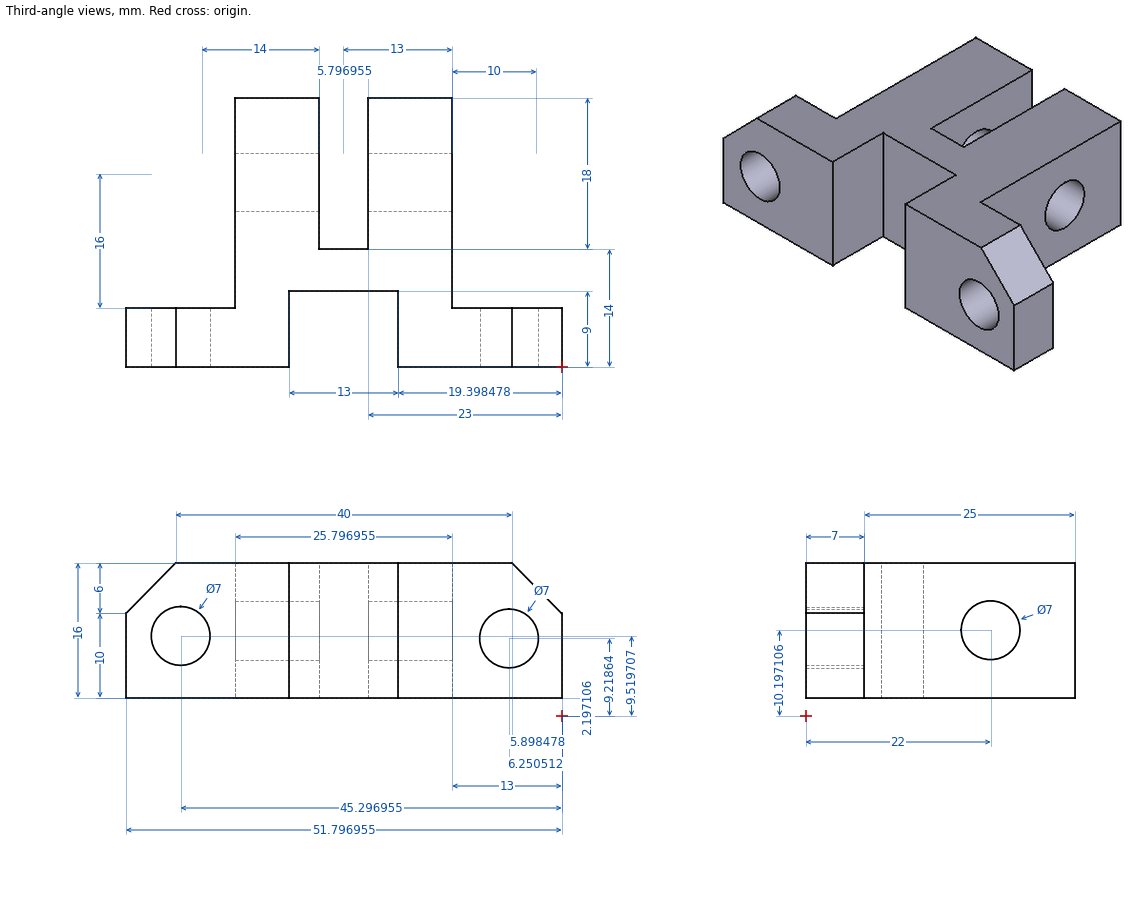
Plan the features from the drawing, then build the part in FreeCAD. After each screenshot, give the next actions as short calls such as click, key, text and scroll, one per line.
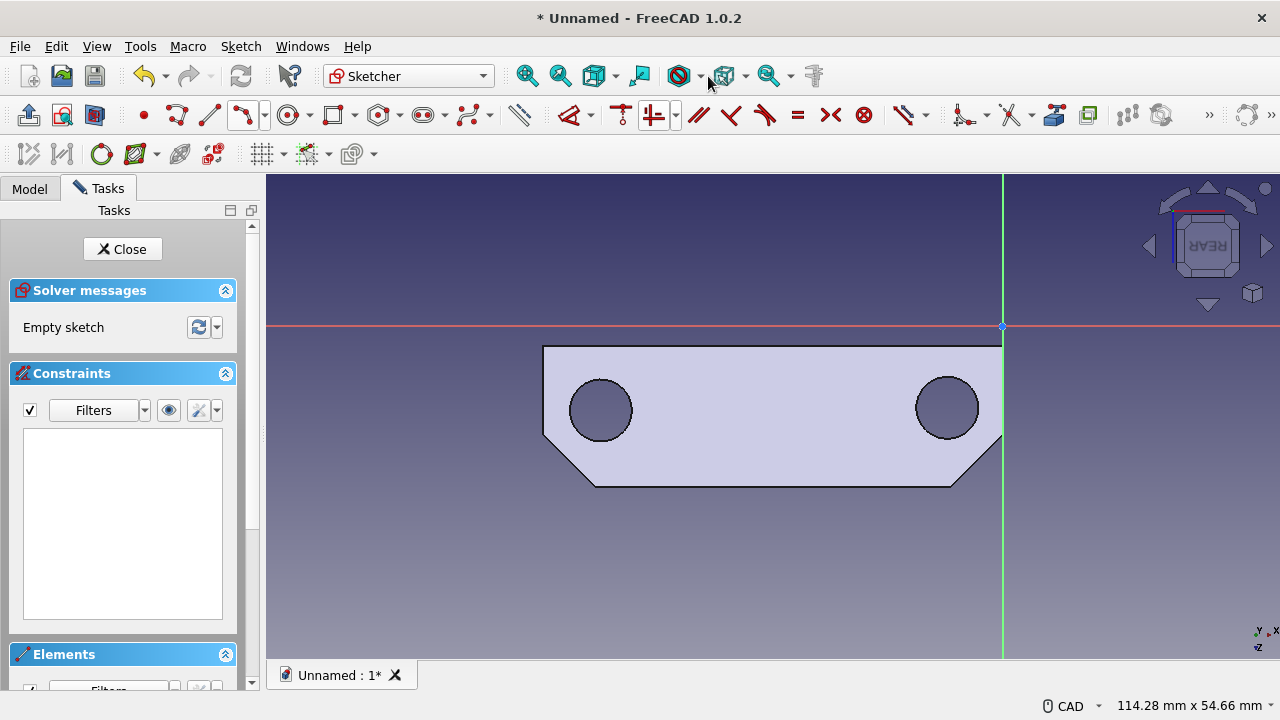
scroll(984, 395, up, 3)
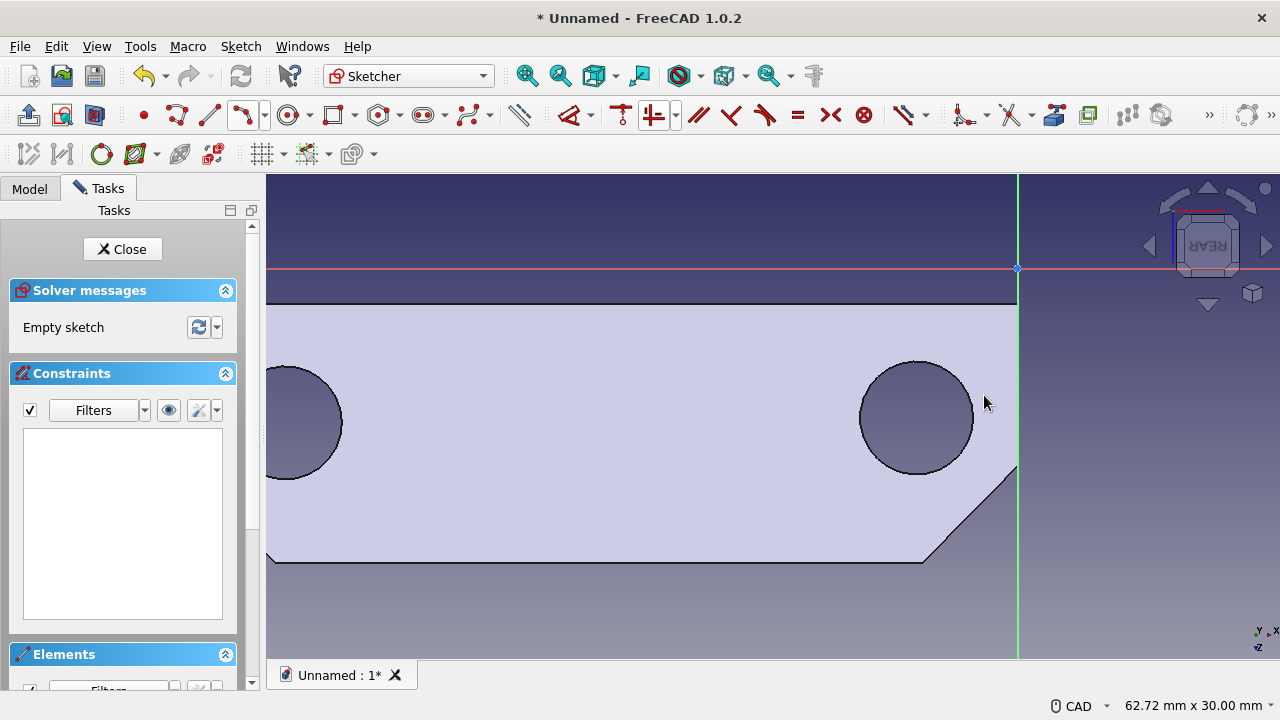
key(g)
key(r)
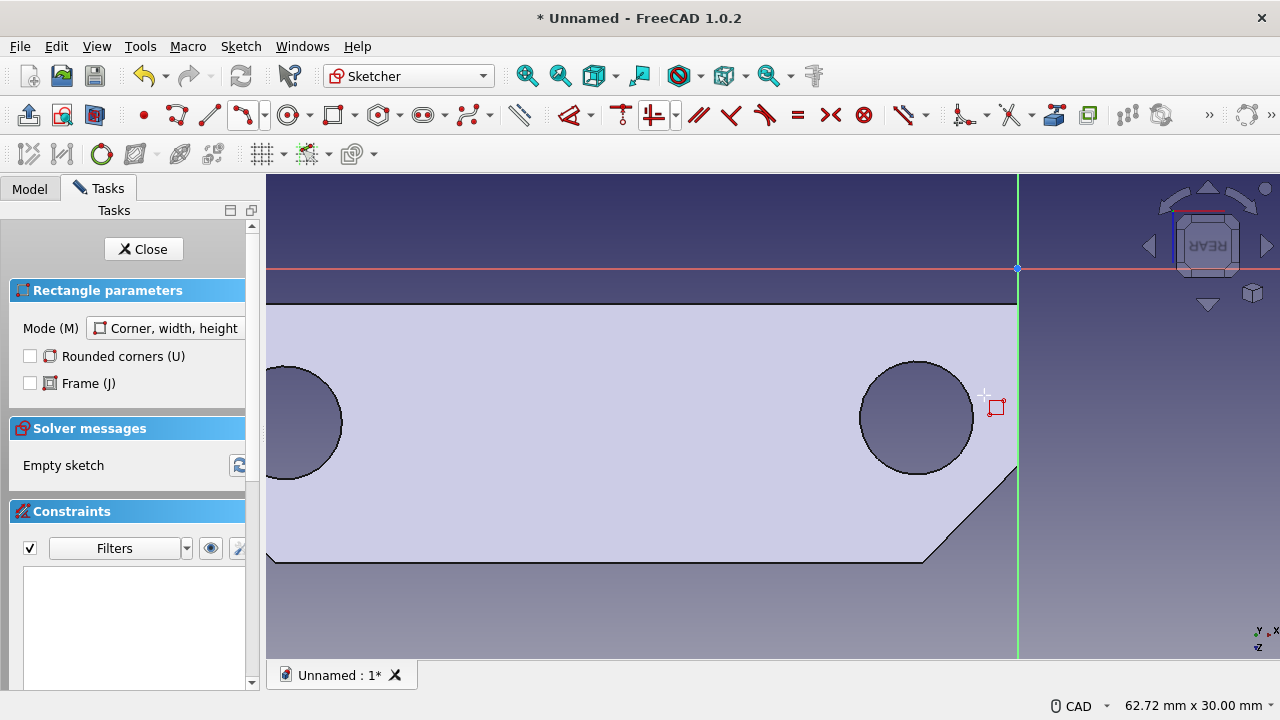
click(390, 304)
click(807, 563)
key(Escape)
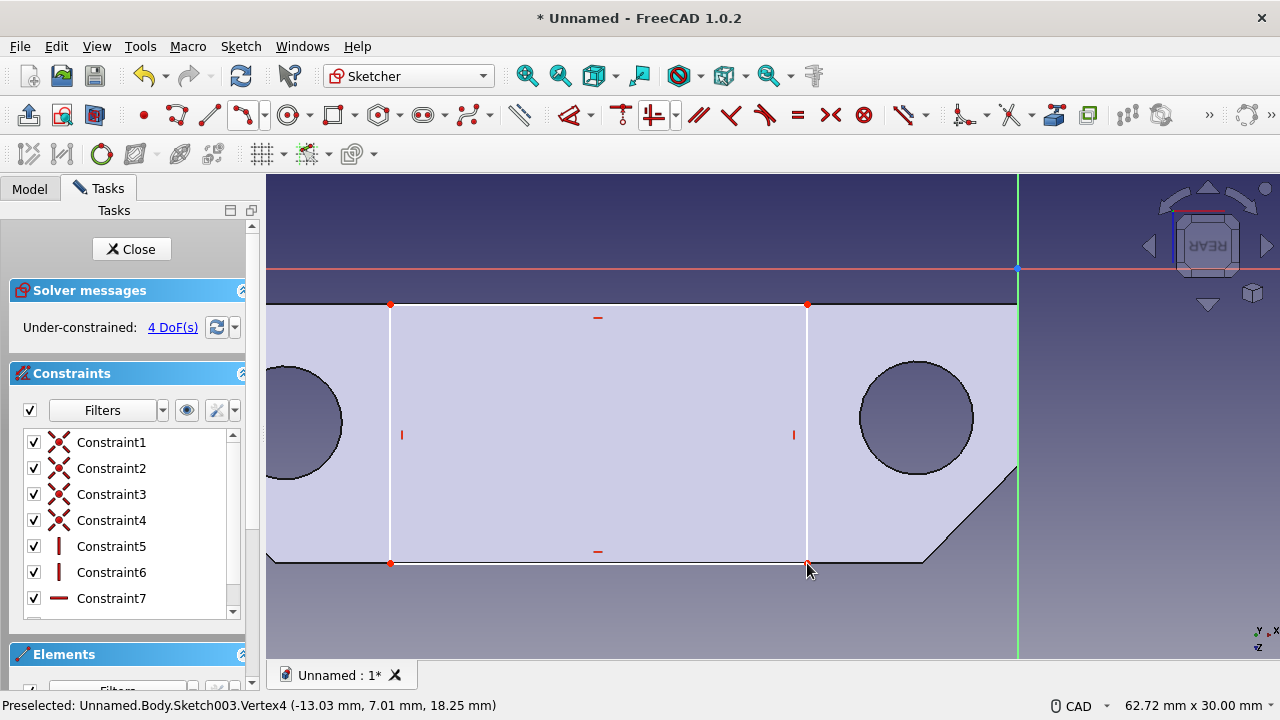
key(d)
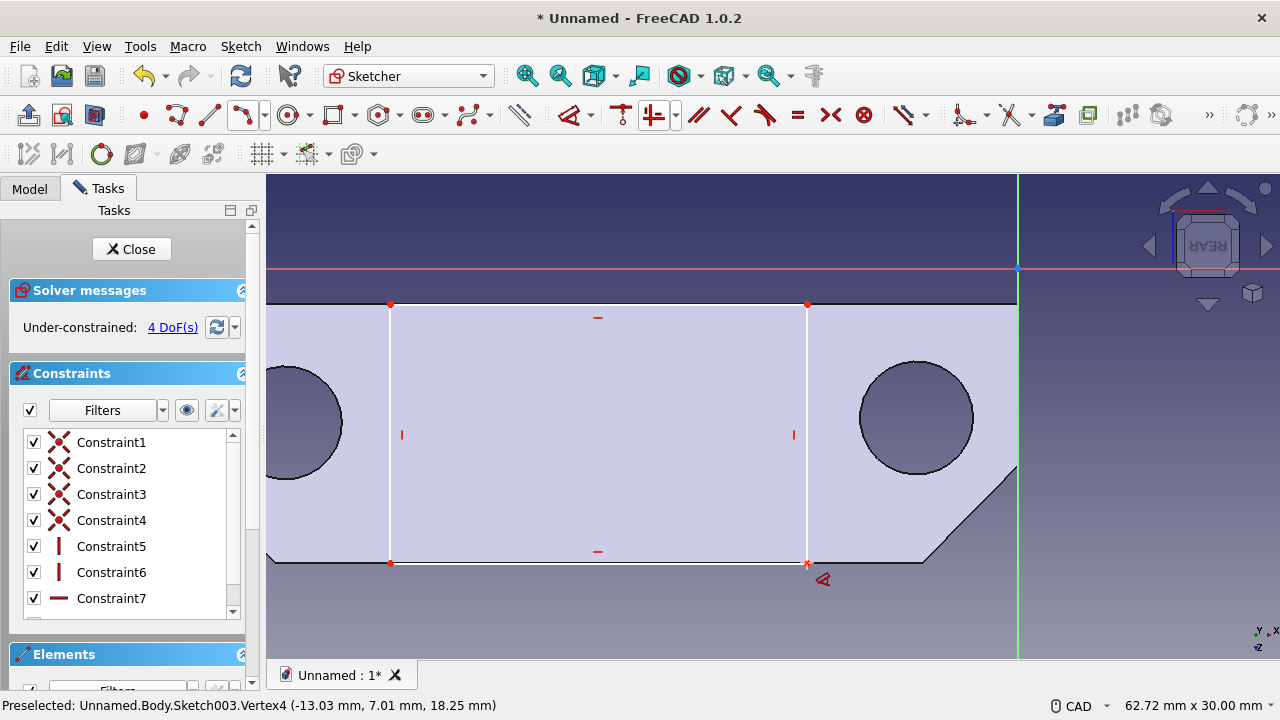
click(390, 383)
click(356, 435)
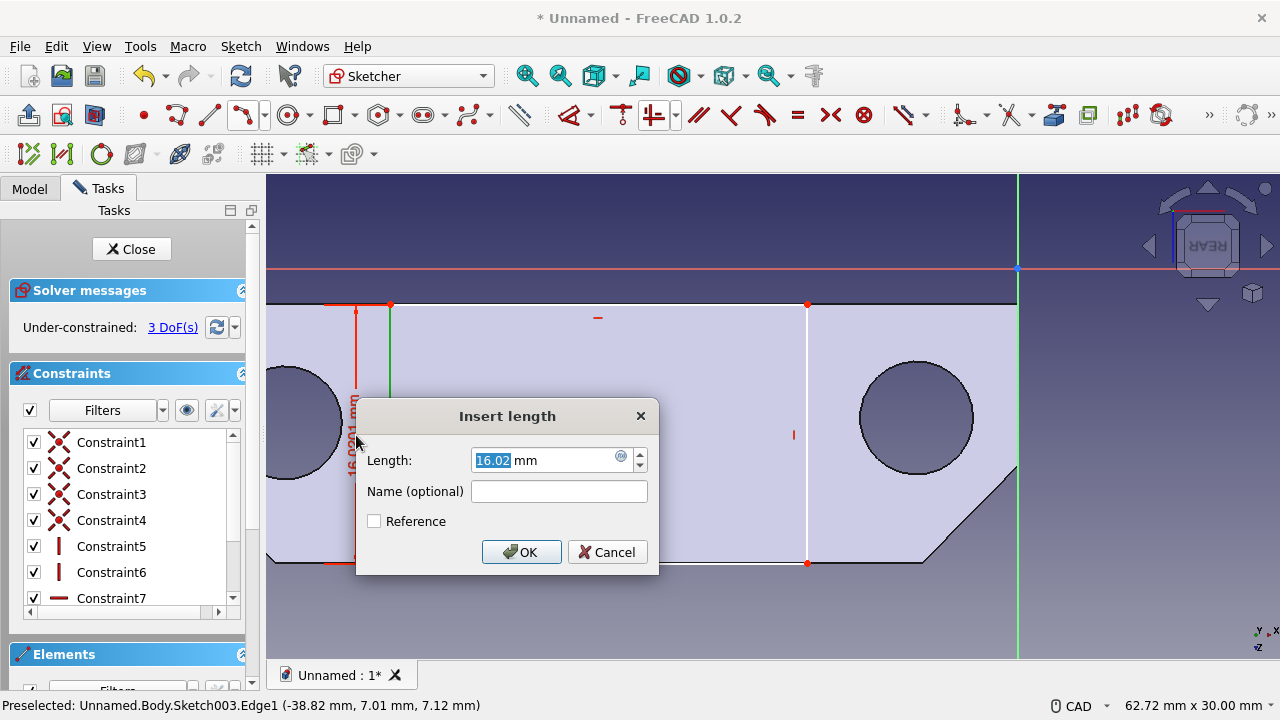
text(16)
key(Return)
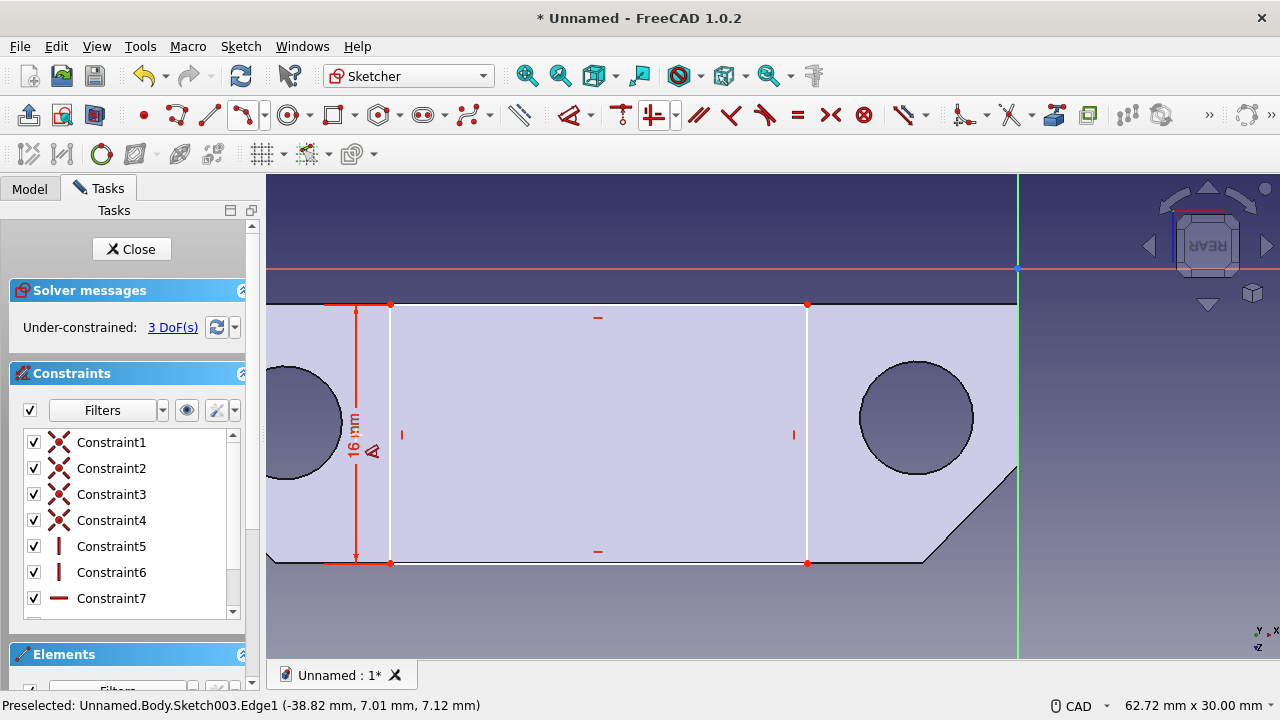
click(807, 564)
click(912, 598)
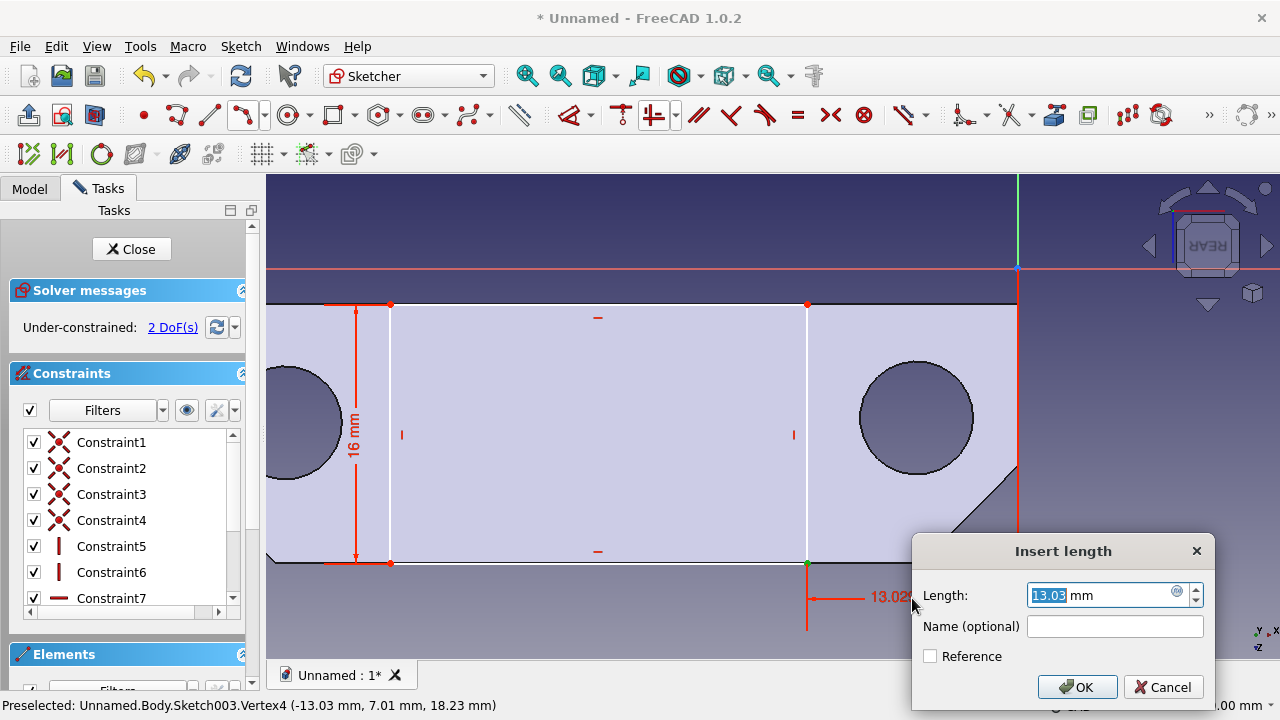
text(13)
key(Return)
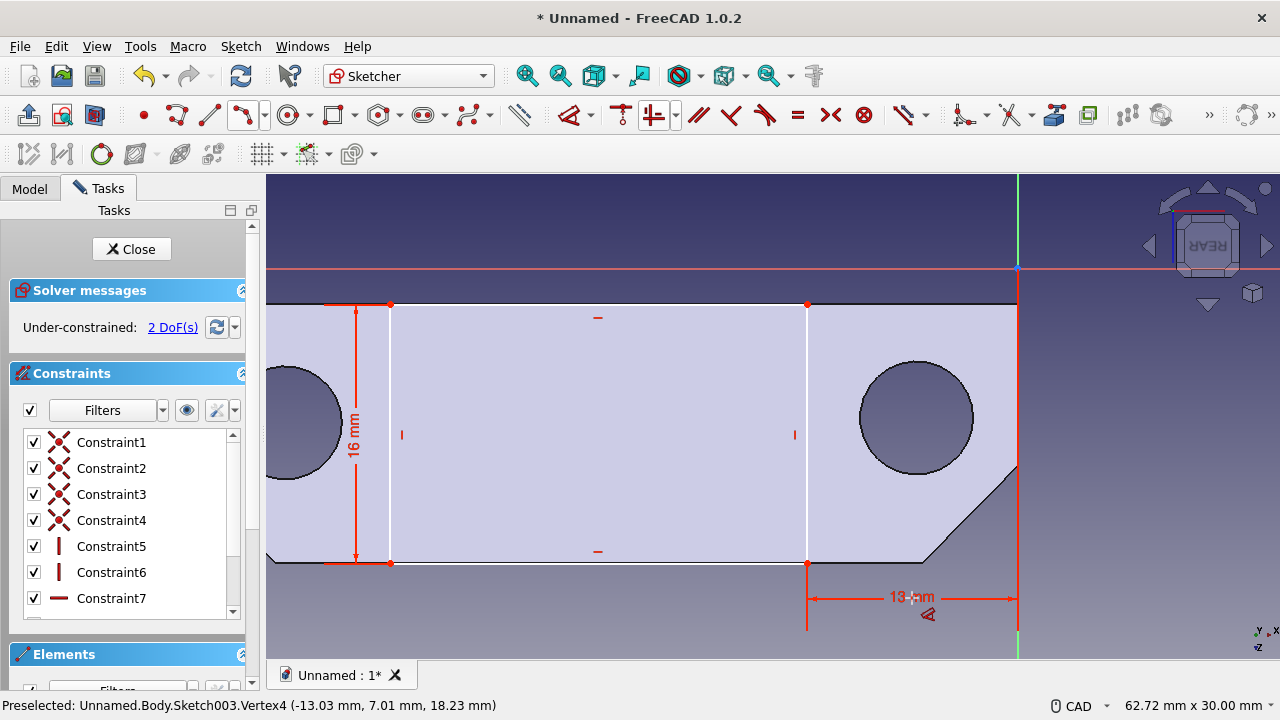
click(515, 564)
click(599, 598)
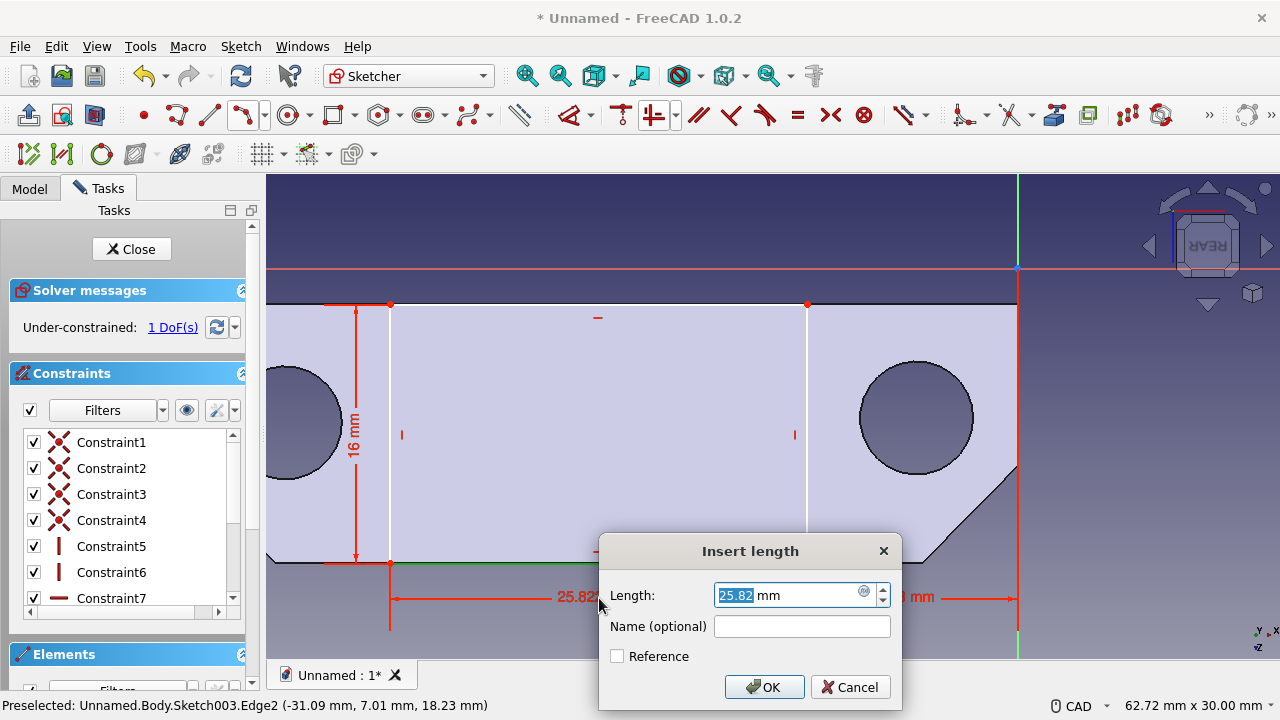
text(25.796955)
key(Return)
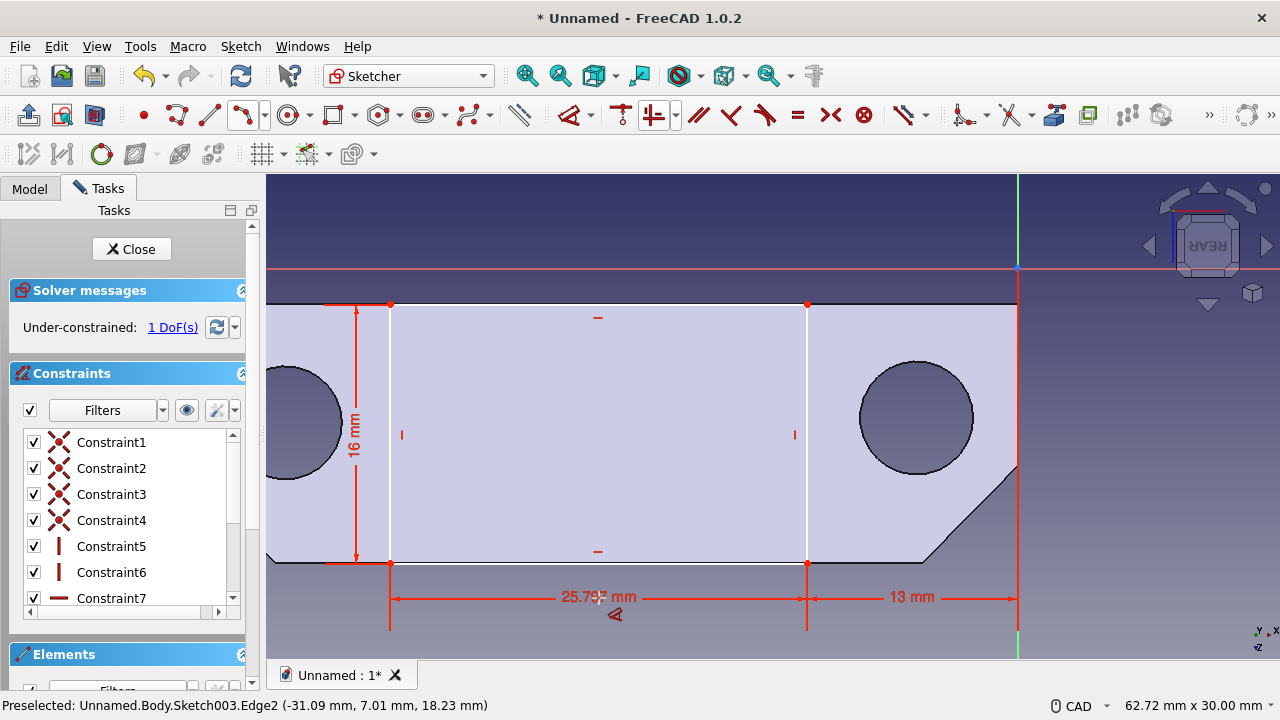
click(390, 305)
click(1052, 287)